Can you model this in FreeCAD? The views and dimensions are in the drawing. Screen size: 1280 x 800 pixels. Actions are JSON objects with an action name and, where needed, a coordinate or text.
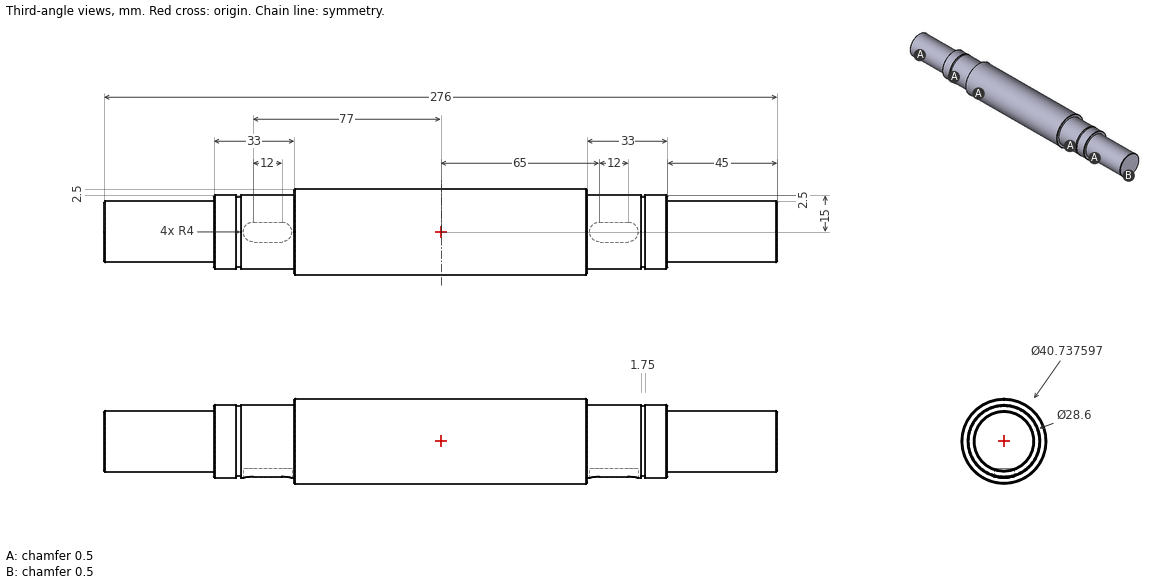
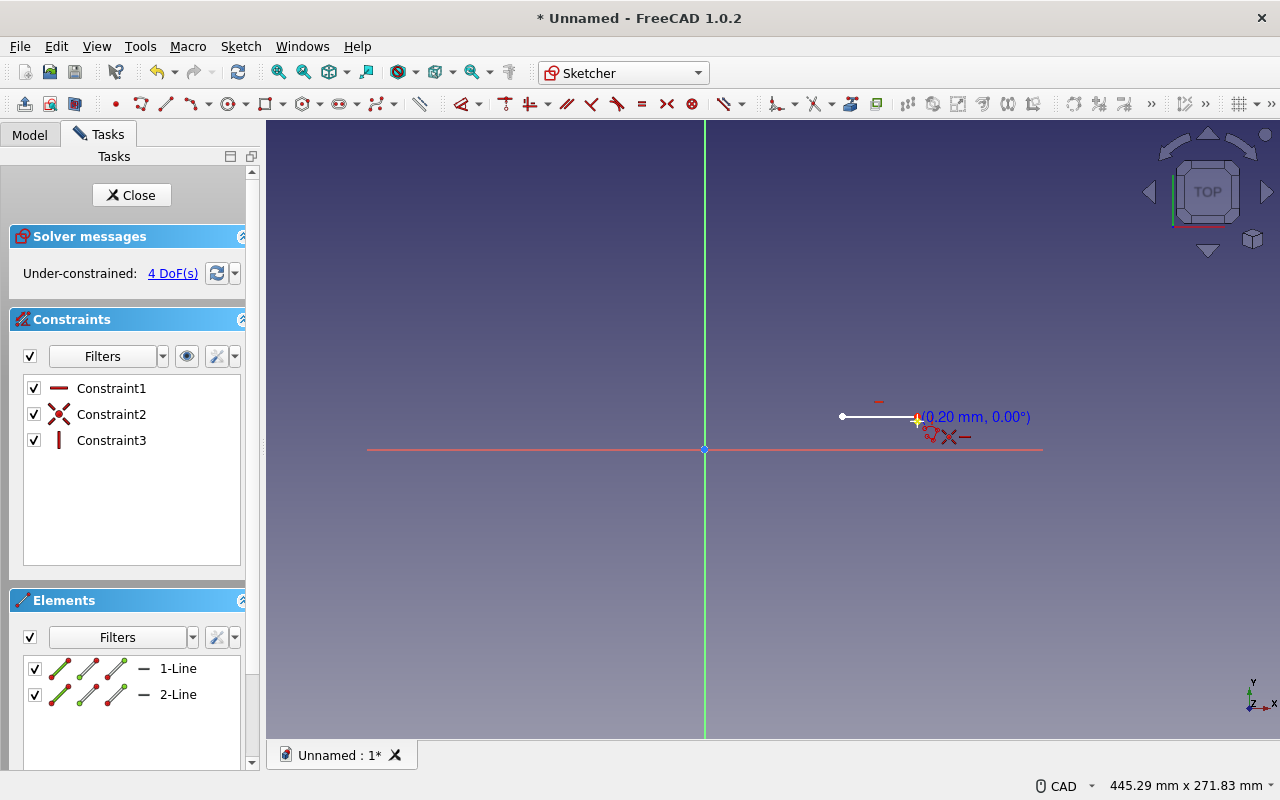
{"action": "left_click", "coordinate": [1019, 421]}
{"action": "left_click", "coordinate": [1019, 450]}
{"action": "left_click", "coordinate": [391, 441]}
{"action": "left_click", "coordinate": [391, 421]}
{"action": "left_click", "coordinate": [493, 421]}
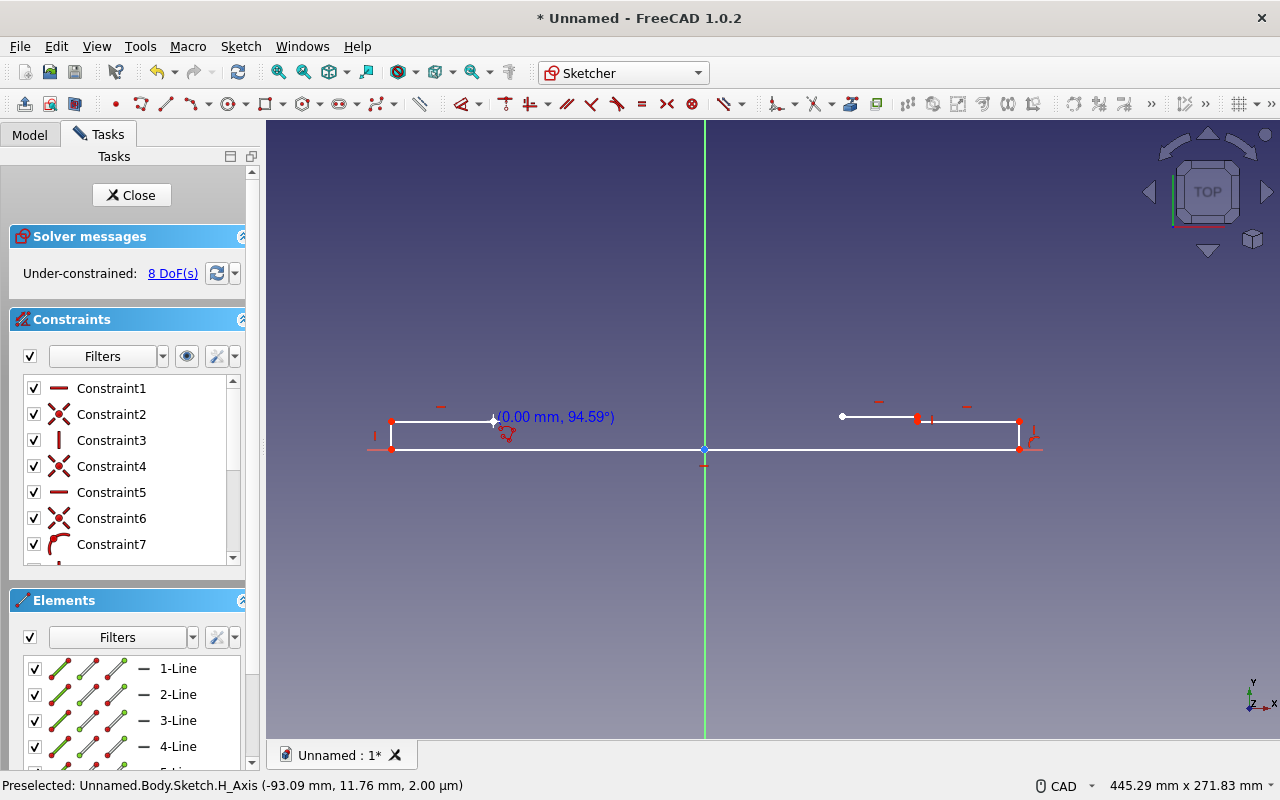
{"action": "scroll", "coordinate": [493, 416], "scroll_direction": "up", "scroll_amount": 6}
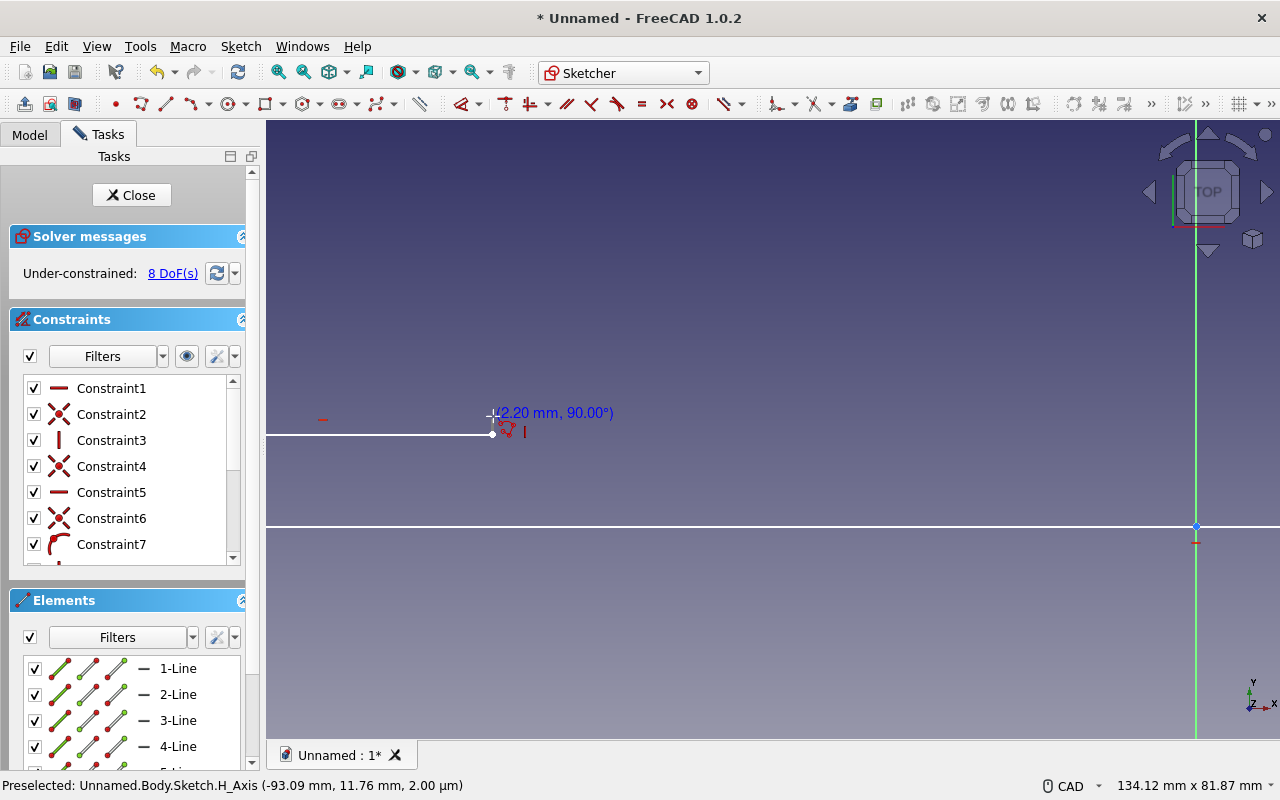
{"action": "left_click", "coordinate": [492, 414]}
{"action": "left_click", "coordinate": [743, 414]}
{"action": "left_click", "coordinate": [743, 395]}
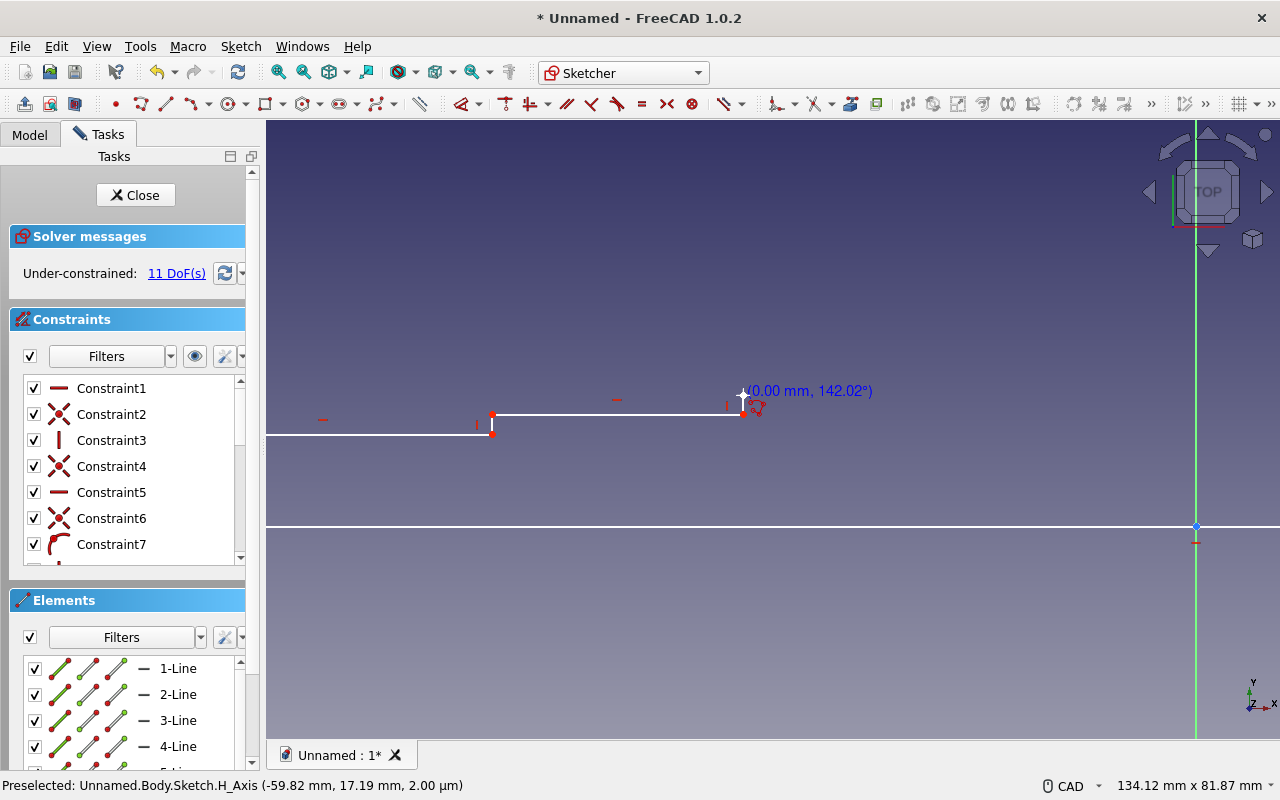
{"action": "scroll", "coordinate": [493, 416], "scroll_direction": "down", "scroll_amount": 6}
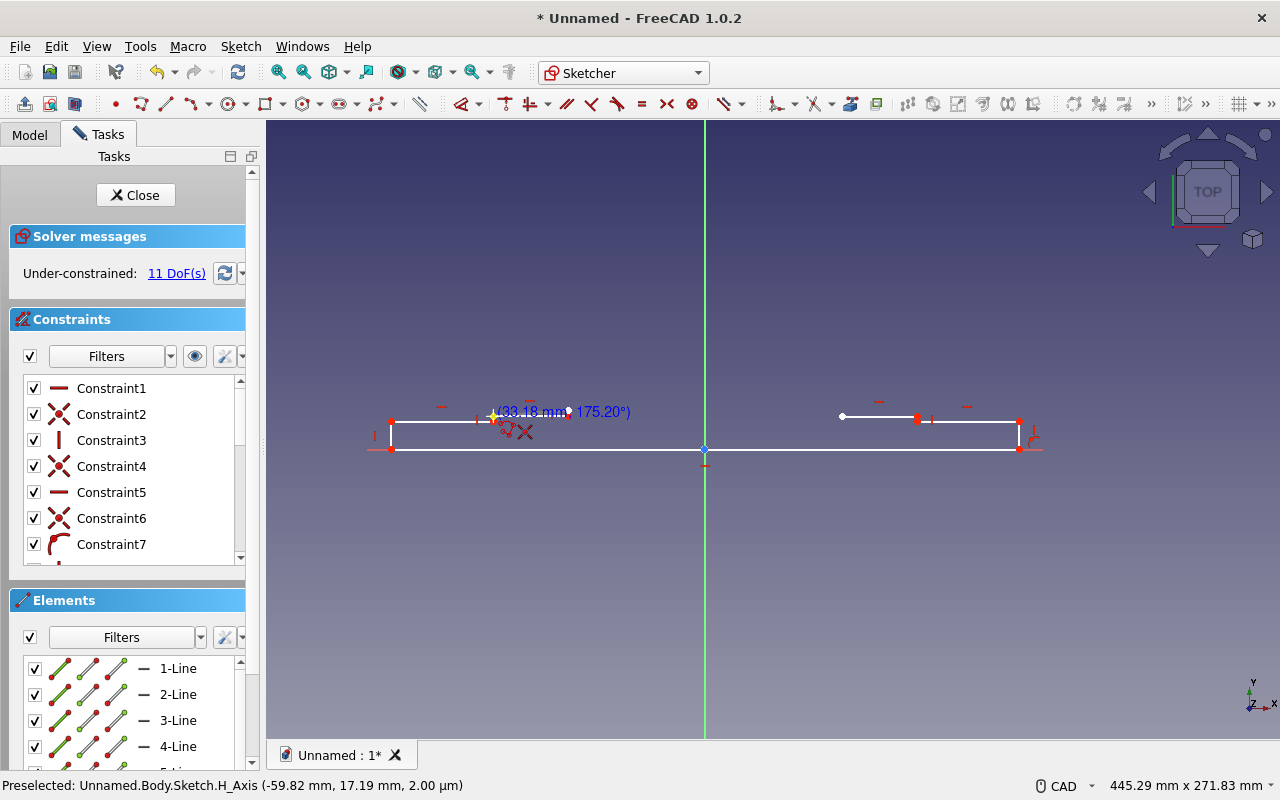
{"action": "scroll", "coordinate": [842, 410], "scroll_direction": "up", "scroll_amount": 6}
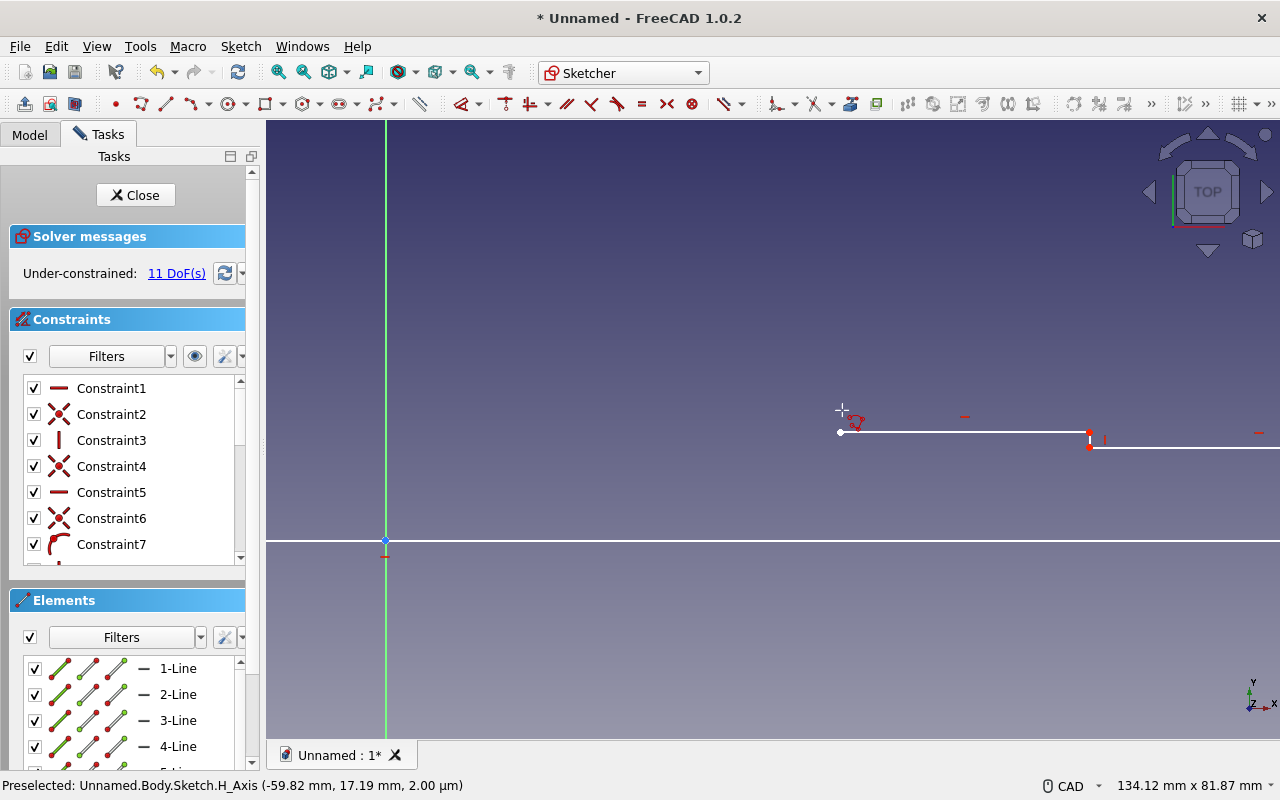
{"action": "left_click", "coordinate": [839, 409]}
{"action": "left_click", "coordinate": [841, 432]}
{"action": "key", "text": "Escape"}
{"action": "key", "text": "Escape"}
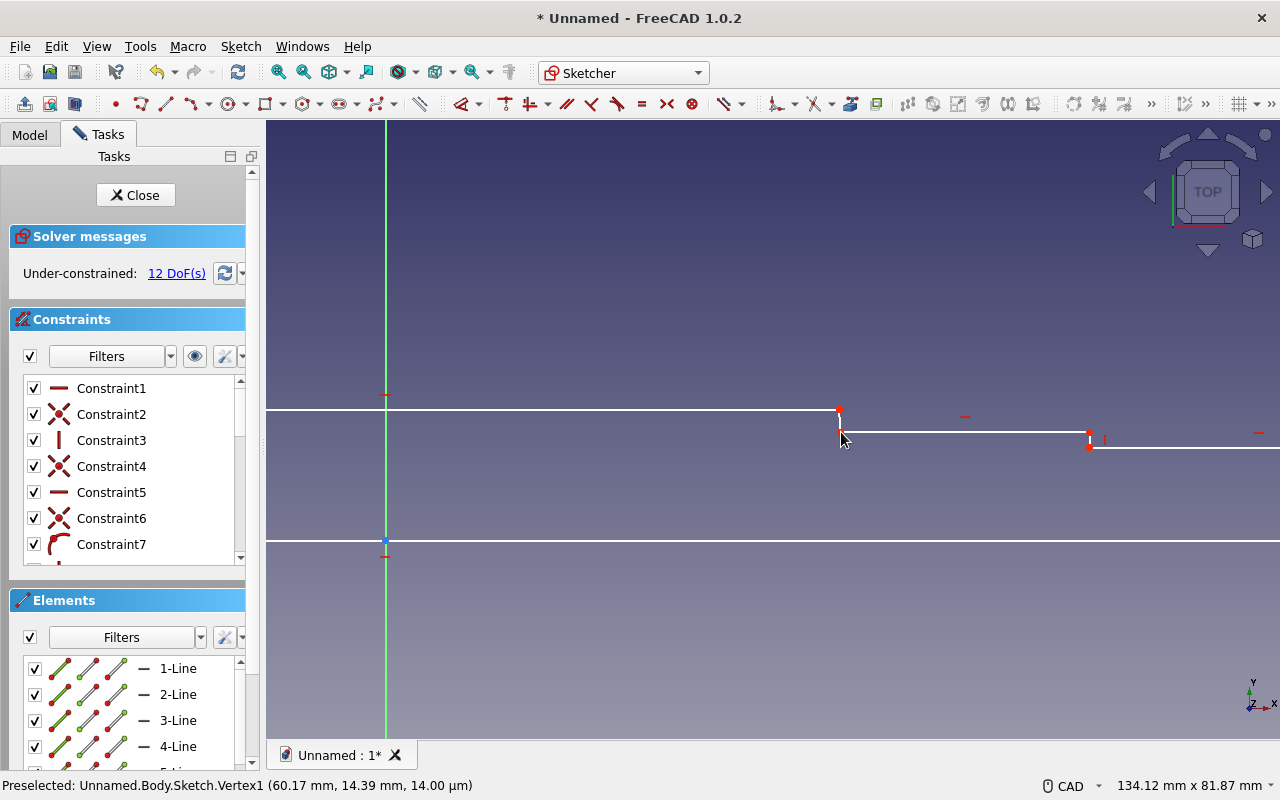
{"action": "scroll", "coordinate": [840, 421], "scroll_direction": "up", "scroll_amount": 2}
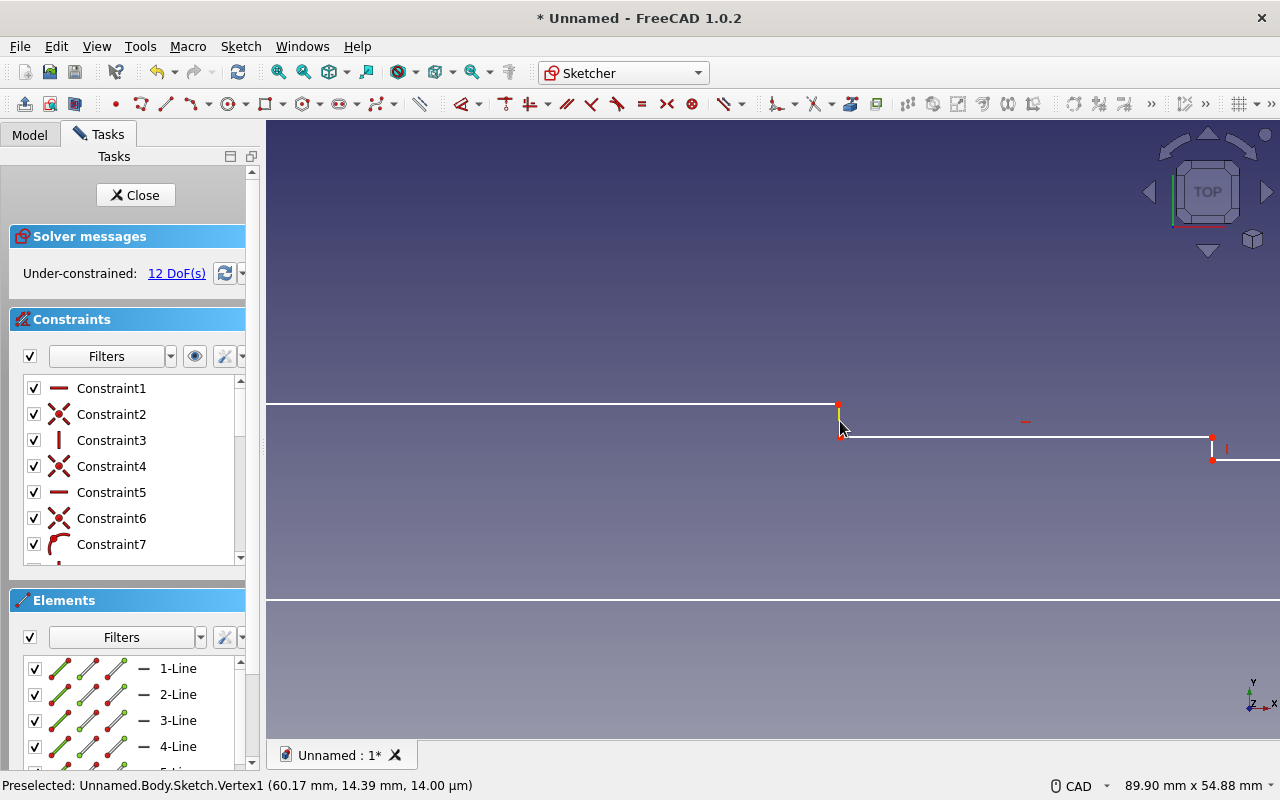
{"action": "left_click", "coordinate": [839, 421]}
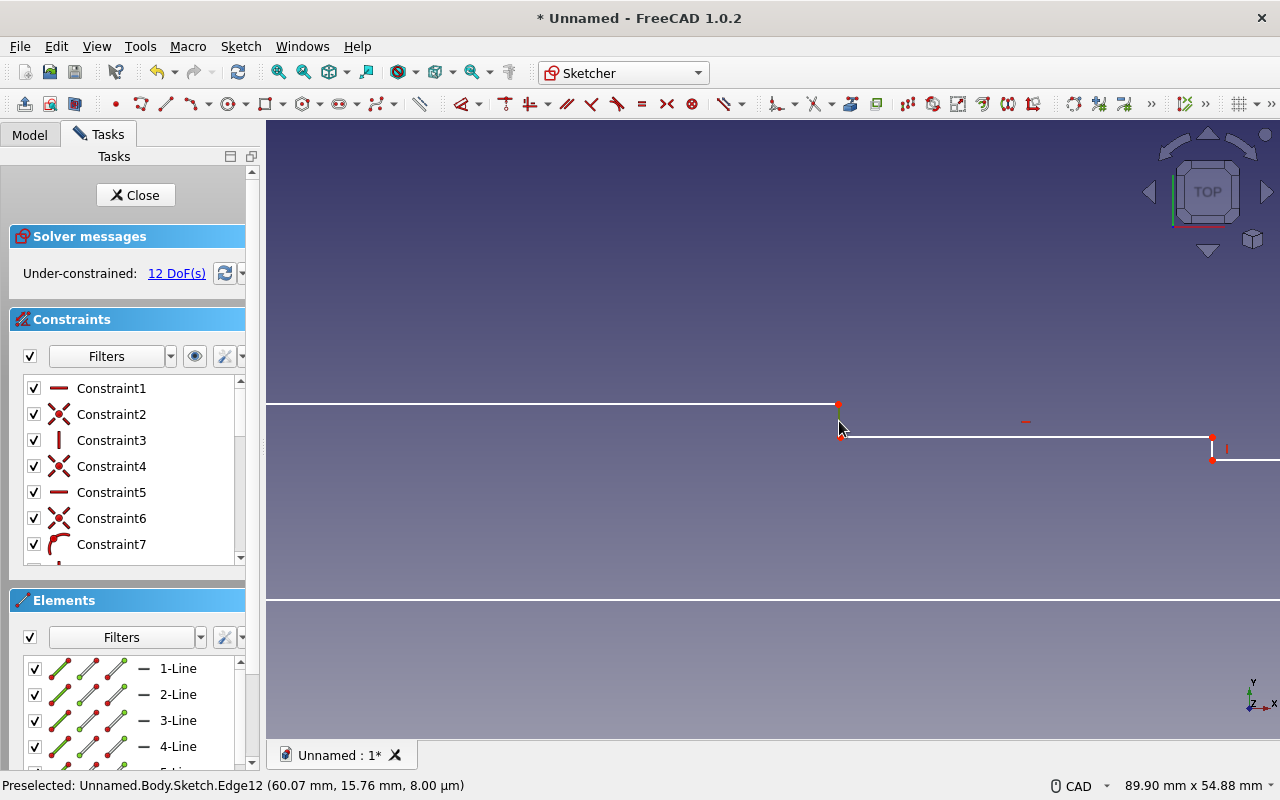
{"action": "left_click", "coordinate": [548, 104]}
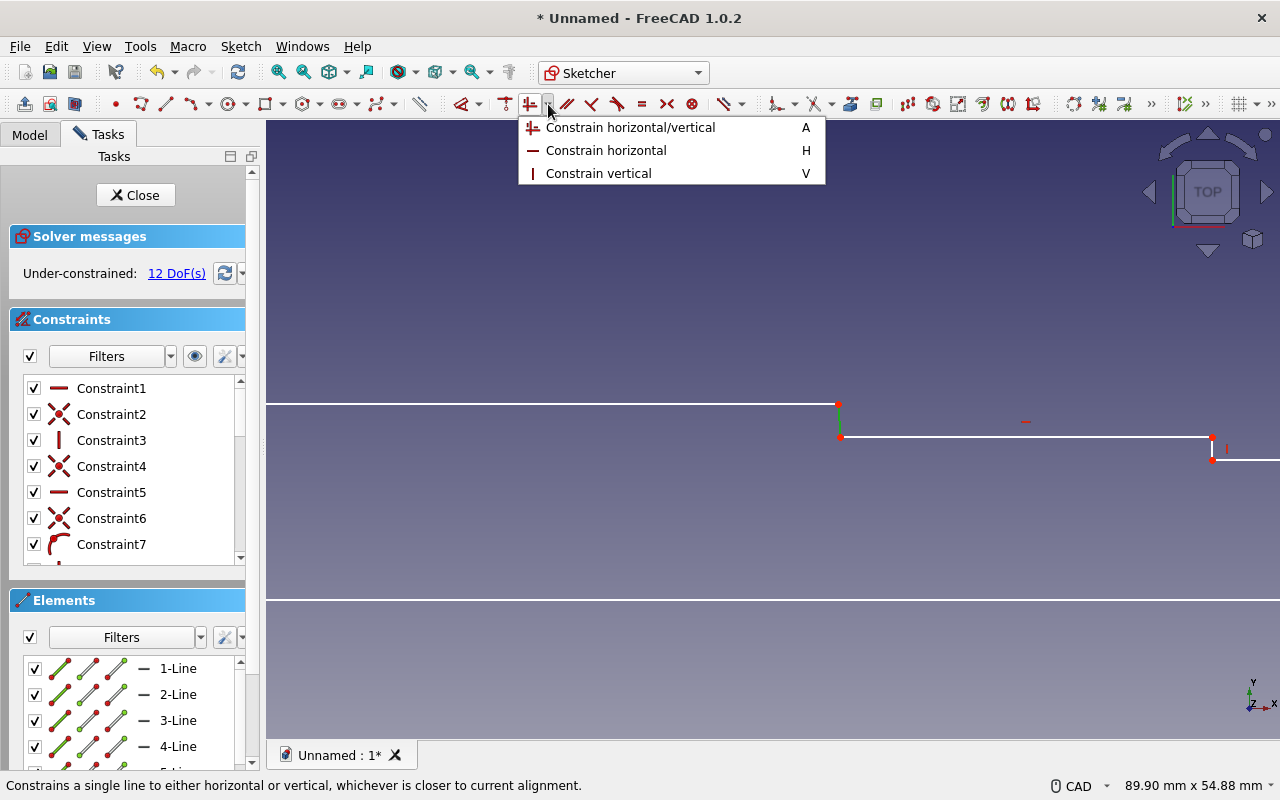
{"action": "left_click", "coordinate": [672, 174]}